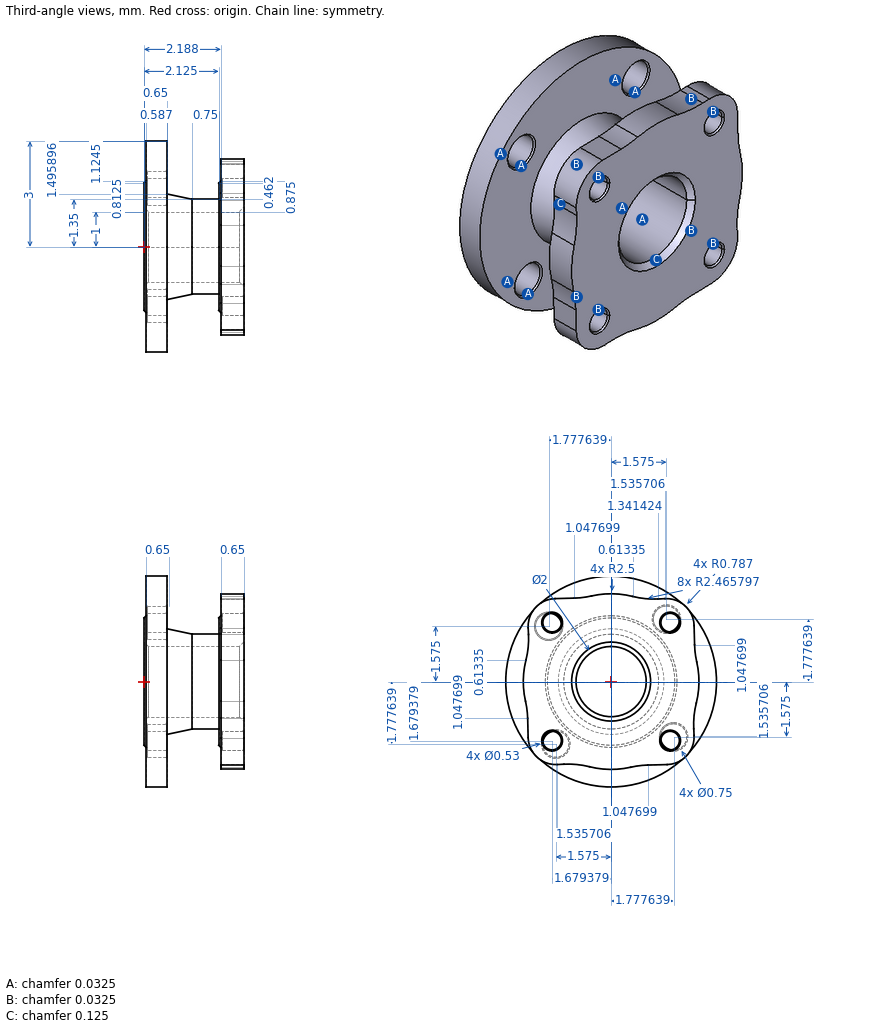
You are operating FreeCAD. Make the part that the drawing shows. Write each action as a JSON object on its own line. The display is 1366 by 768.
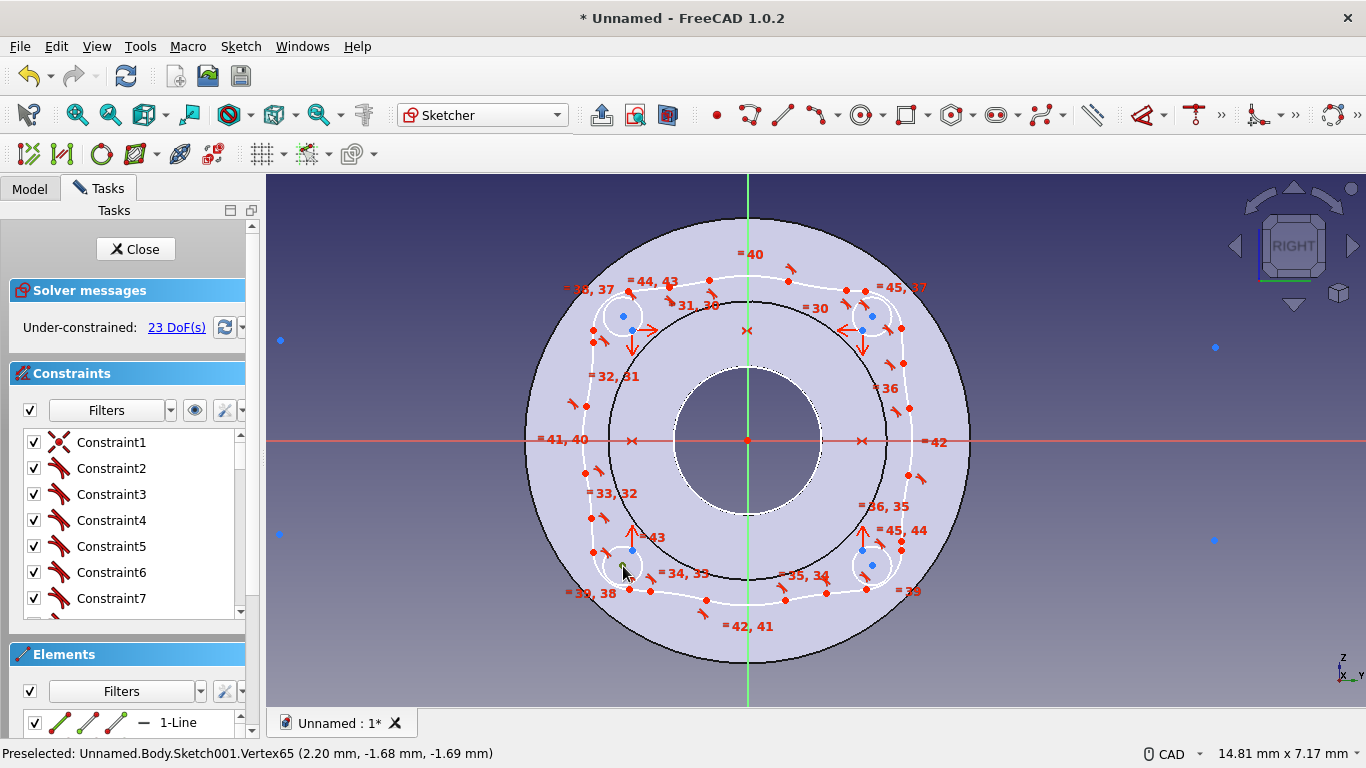
{"action": "left_click", "coordinate": [623, 317]}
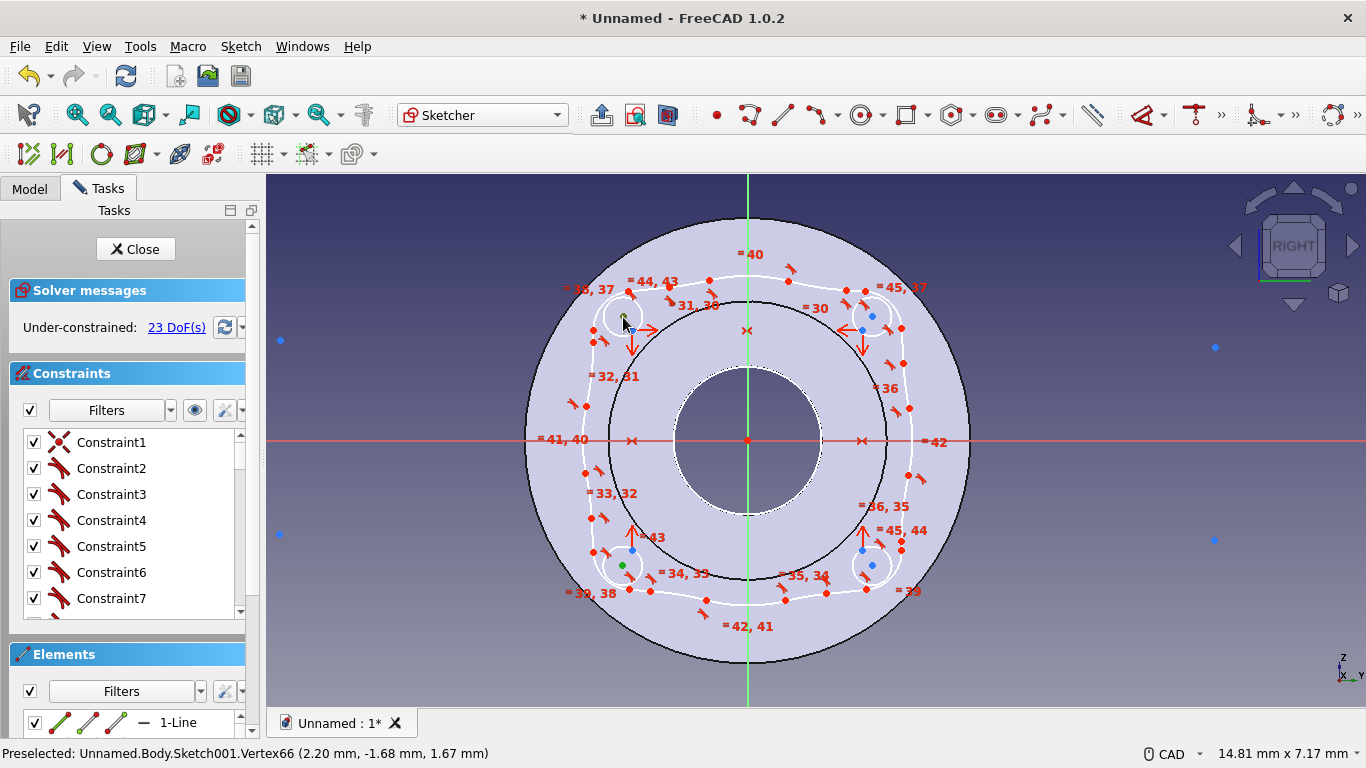
{"action": "left_click", "coordinate": [359, 441]}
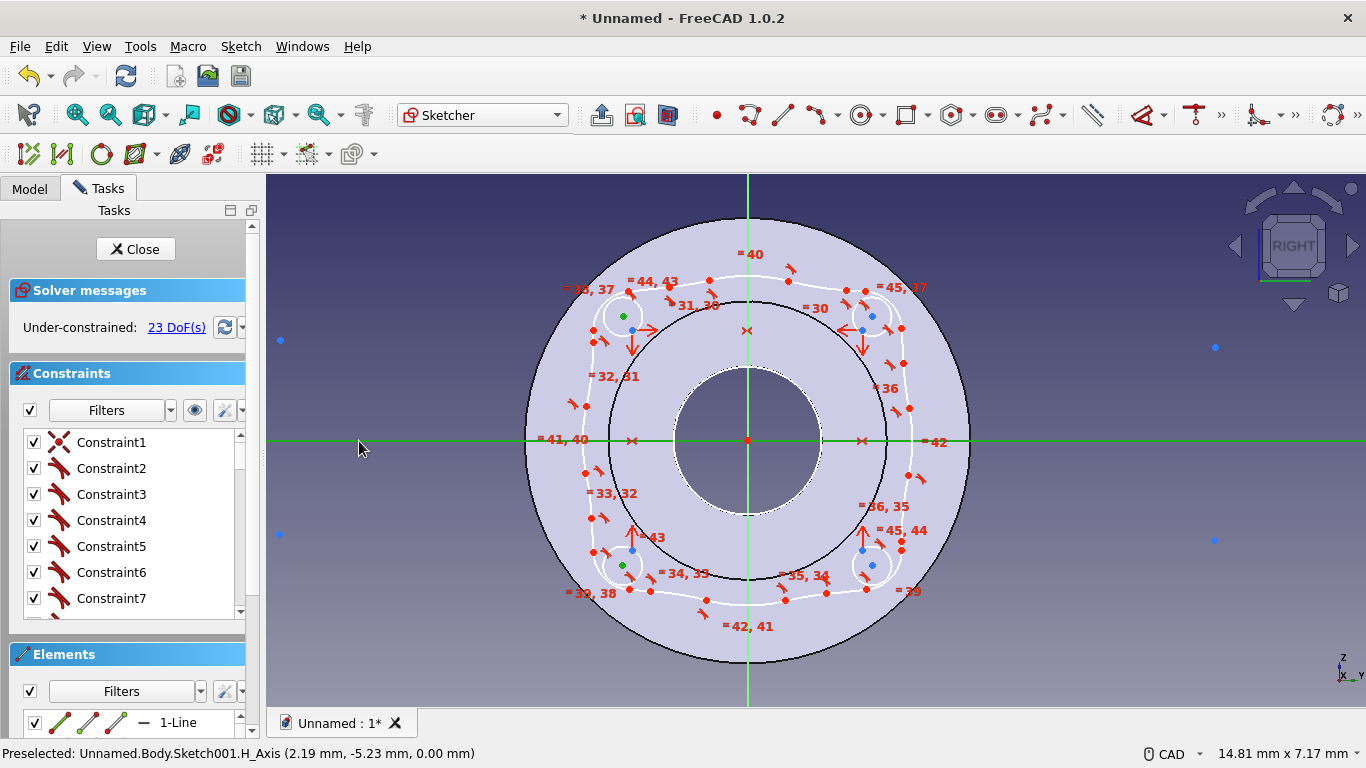
{"action": "key", "text": "s"}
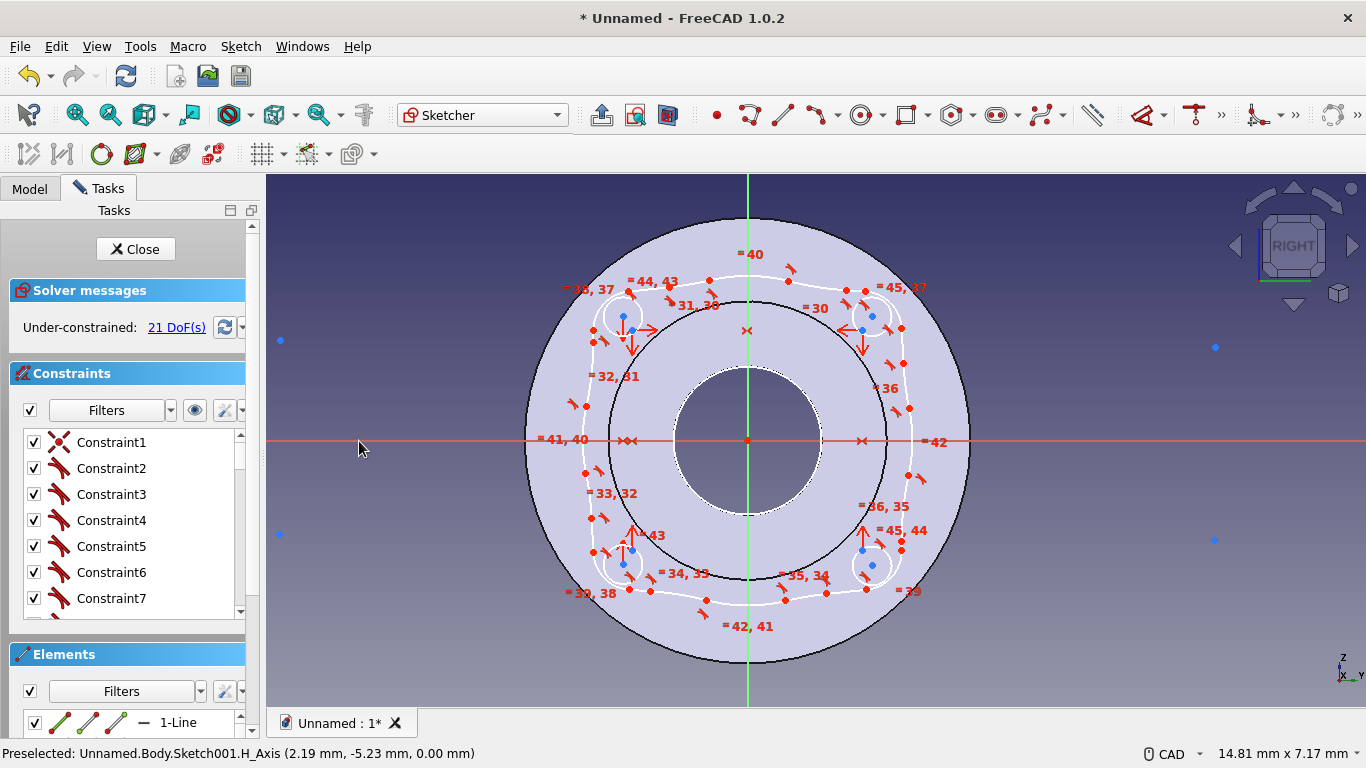
{"action": "left_click", "coordinate": [623, 565]}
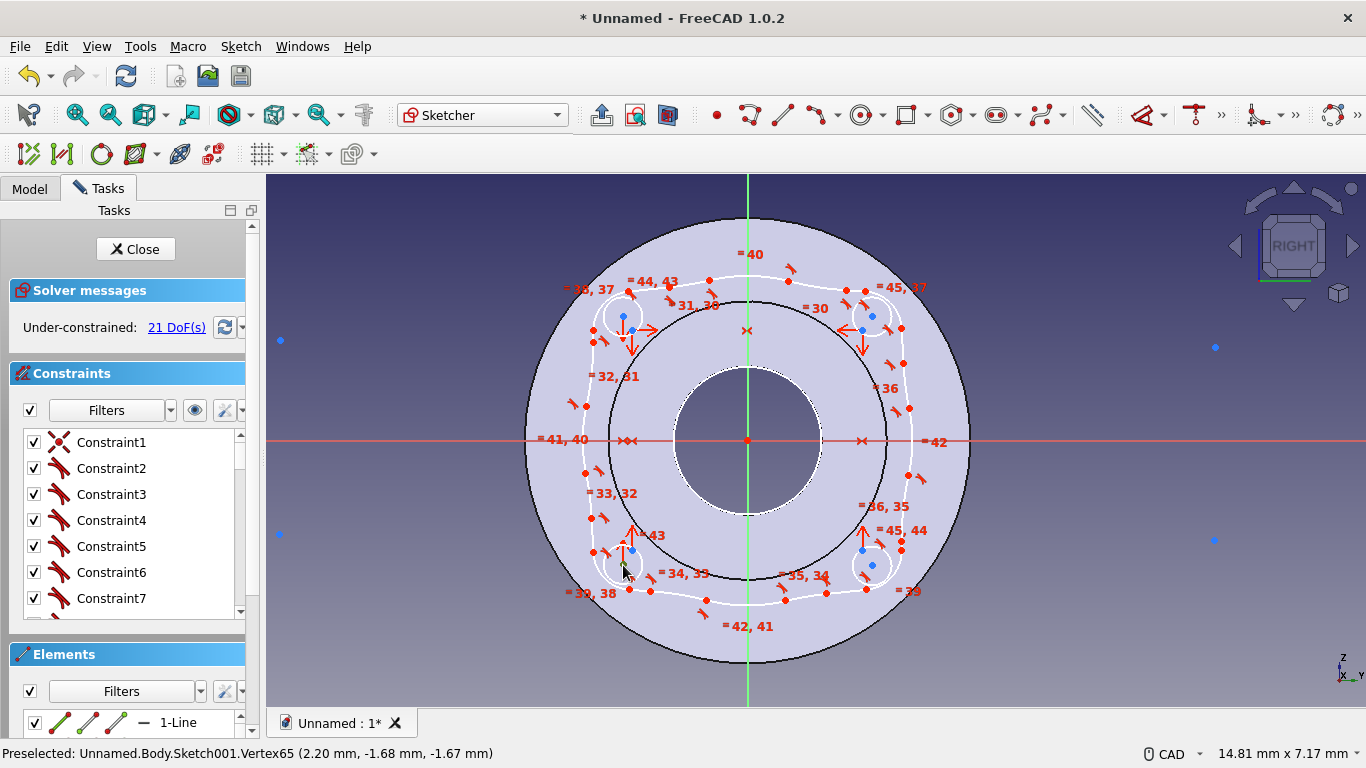
{"action": "left_click", "coordinate": [872, 566]}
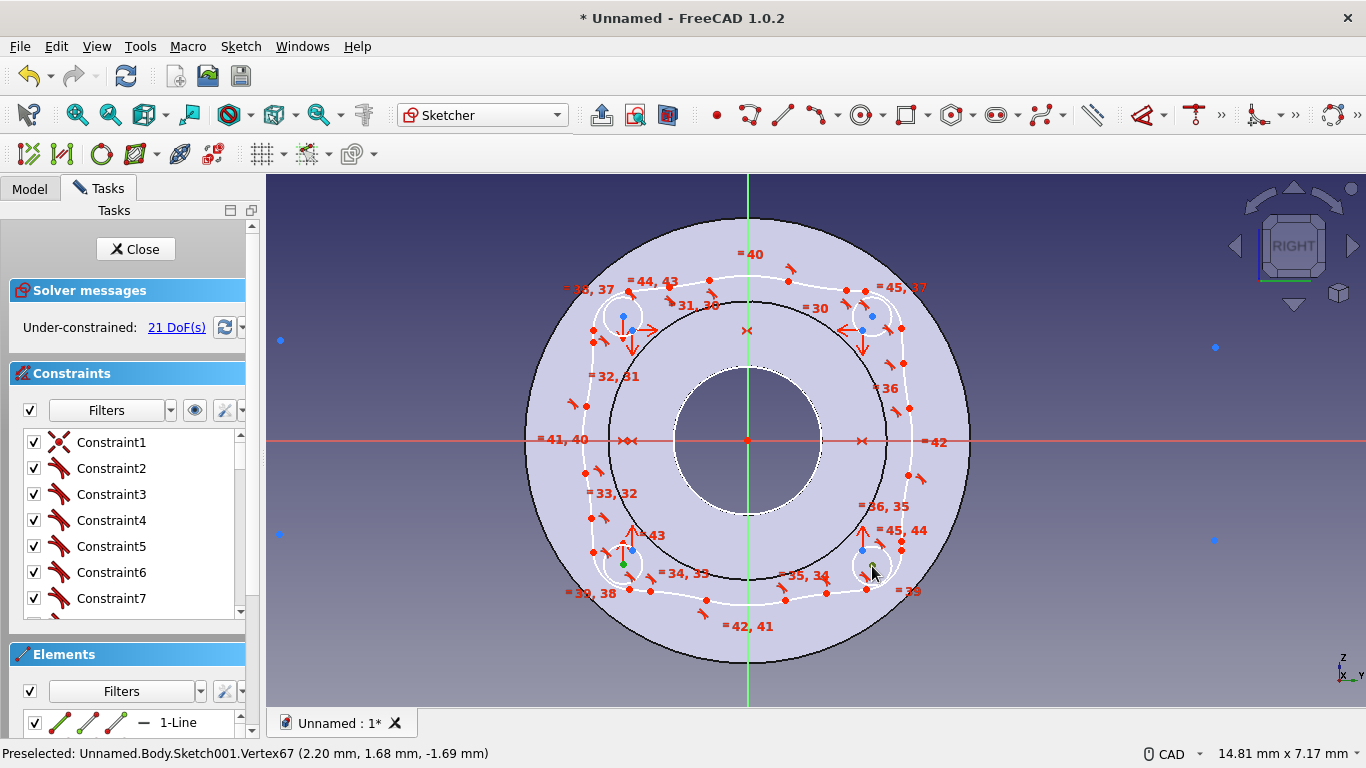
{"action": "left_click", "coordinate": [748, 645]}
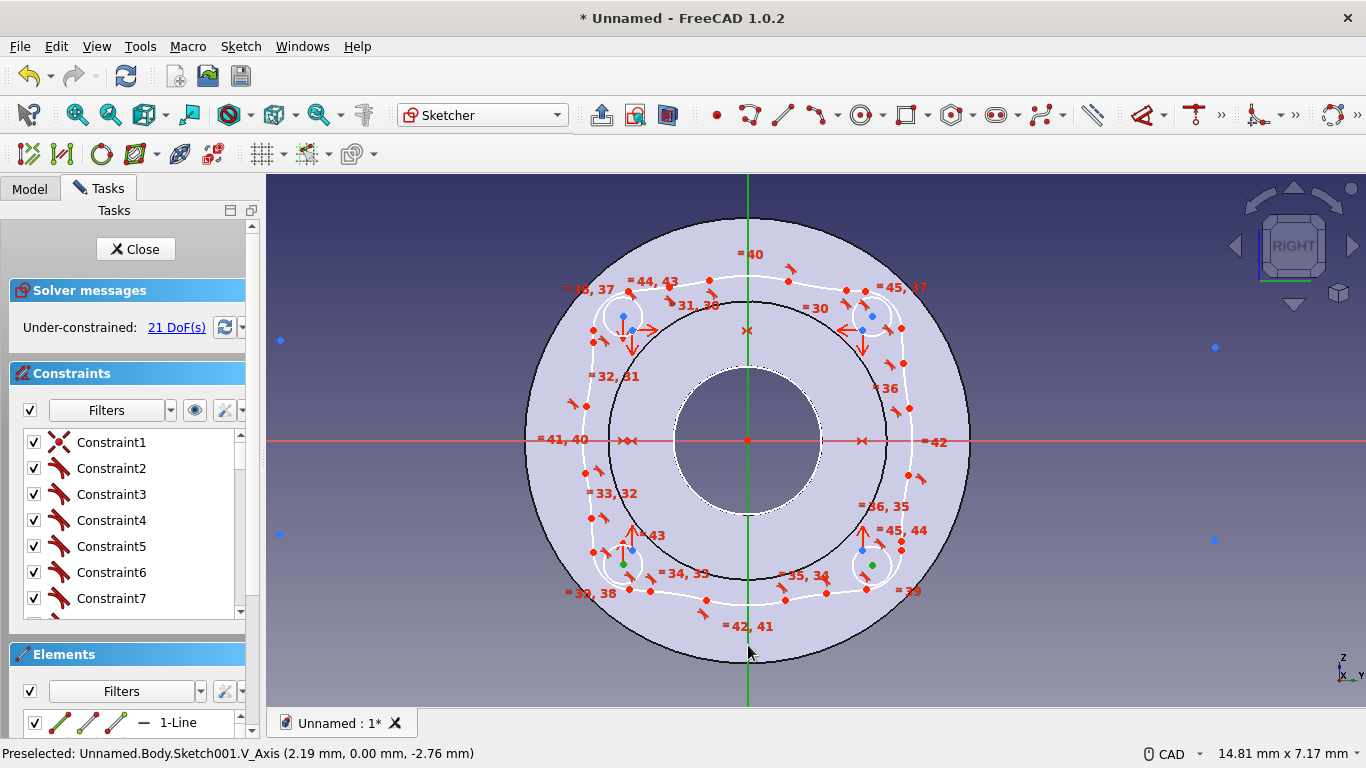
{"action": "key", "text": "s"}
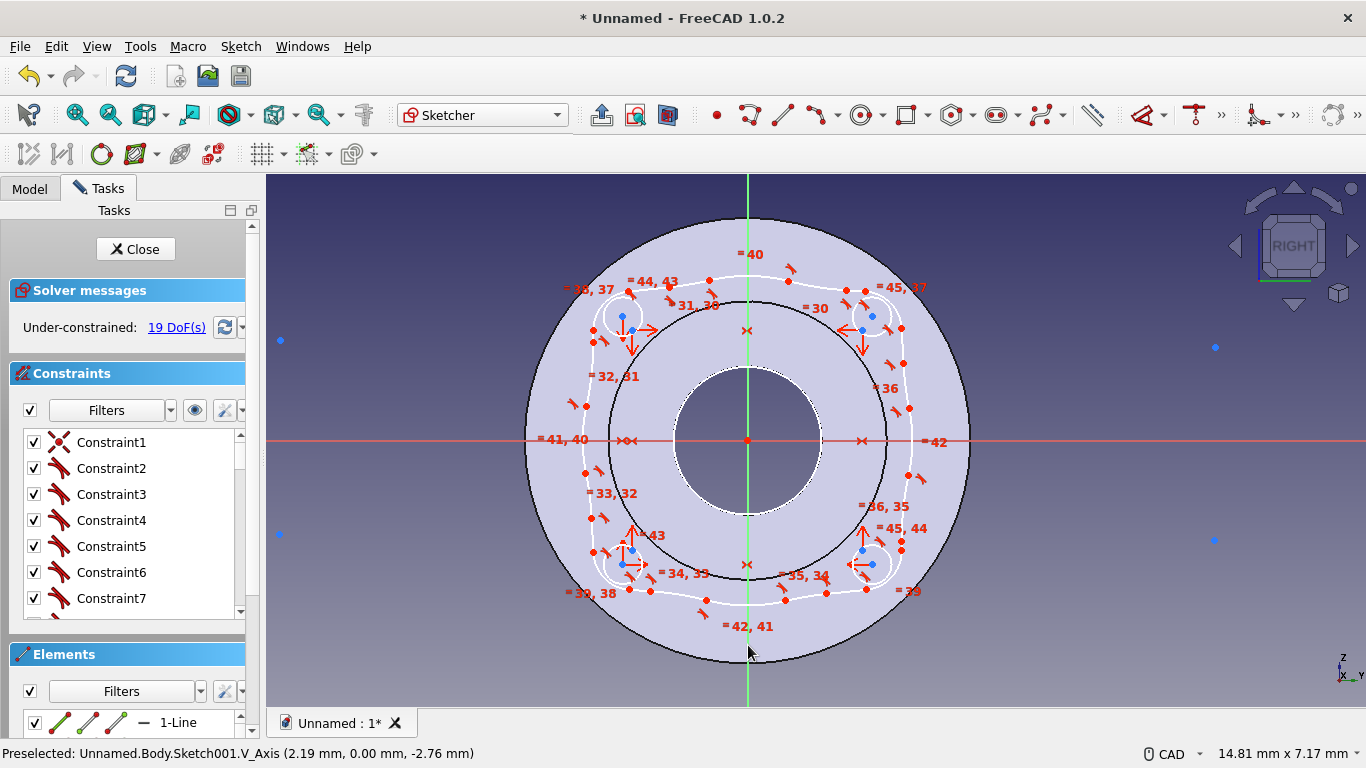
{"action": "left_click", "coordinate": [623, 317]}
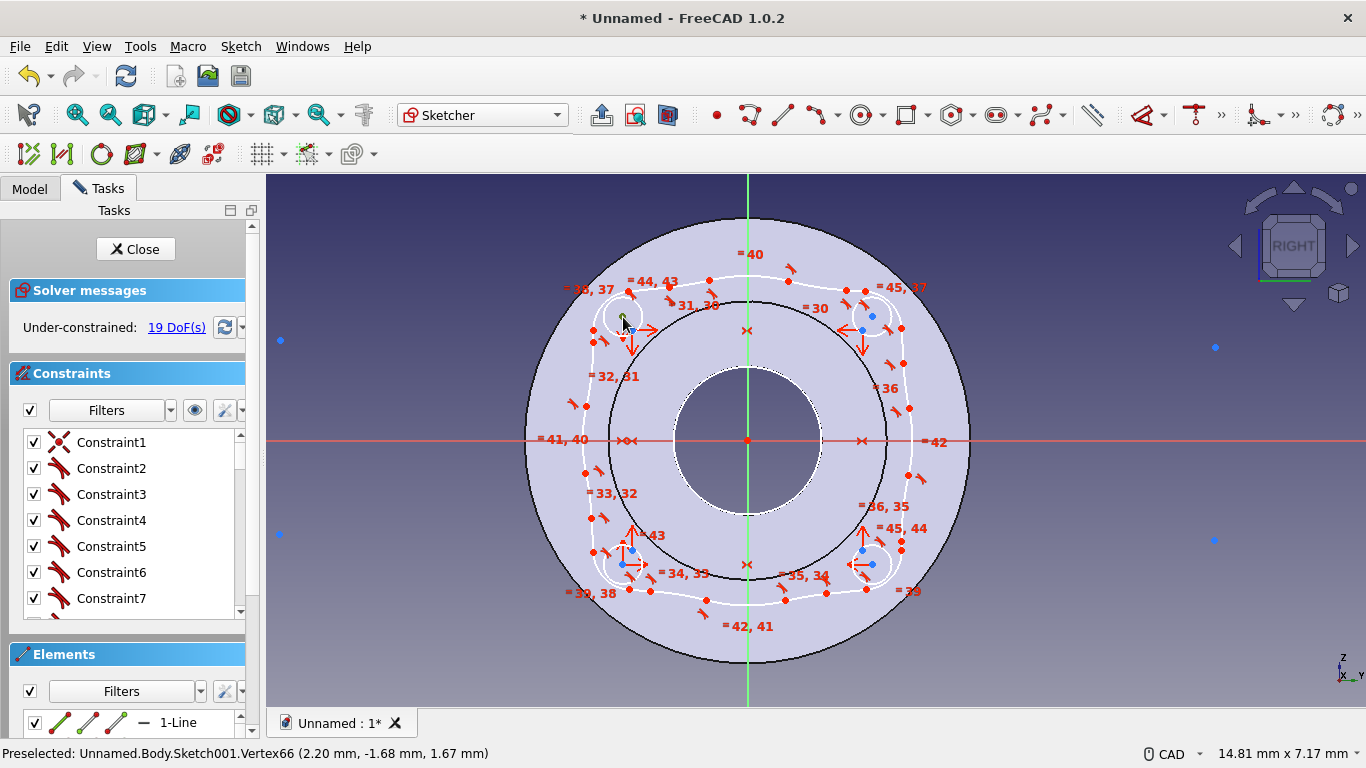
{"action": "left_click", "coordinate": [872, 317]}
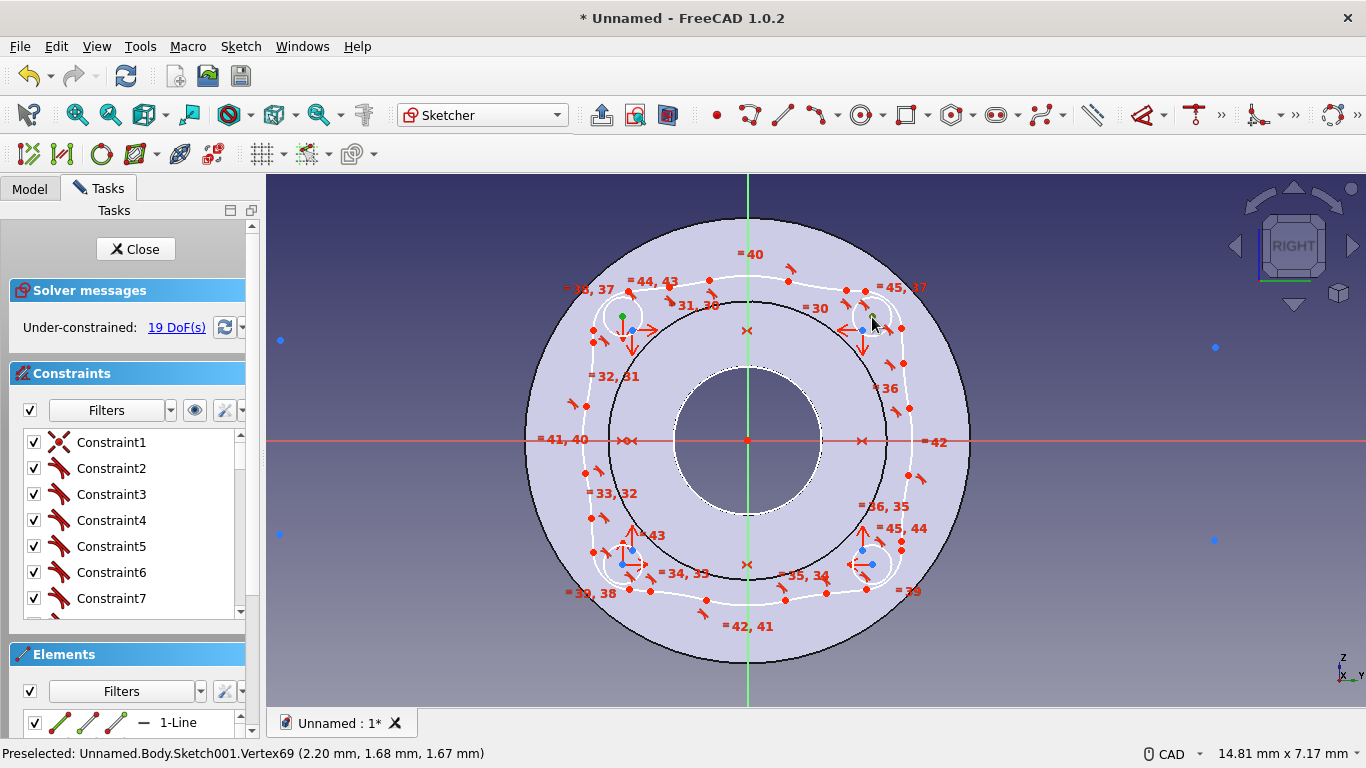
{"action": "left_click", "coordinate": [748, 645]}